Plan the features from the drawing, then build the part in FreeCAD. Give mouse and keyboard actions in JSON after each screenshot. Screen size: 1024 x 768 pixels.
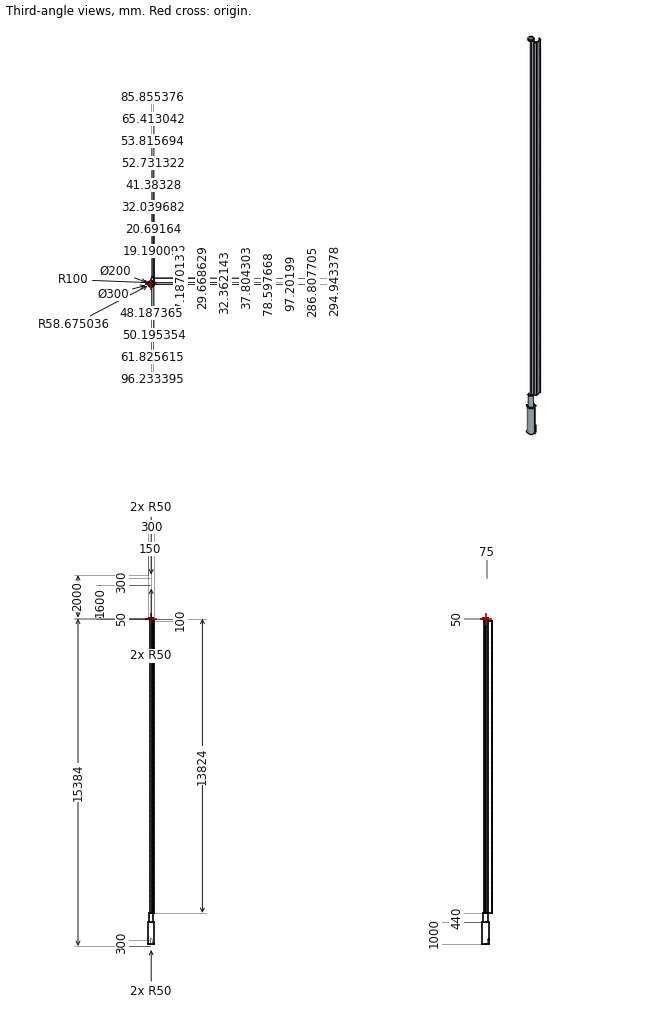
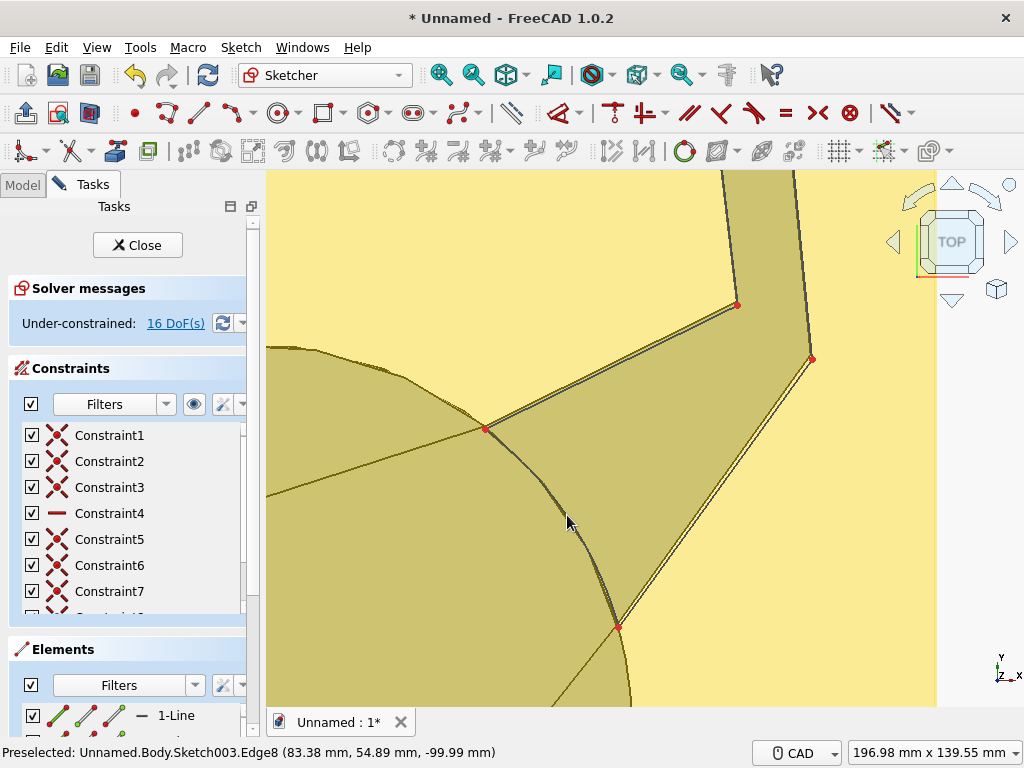
{"action": "scroll", "coordinate": [592, 548], "scroll_direction": "down", "scroll_amount": 7}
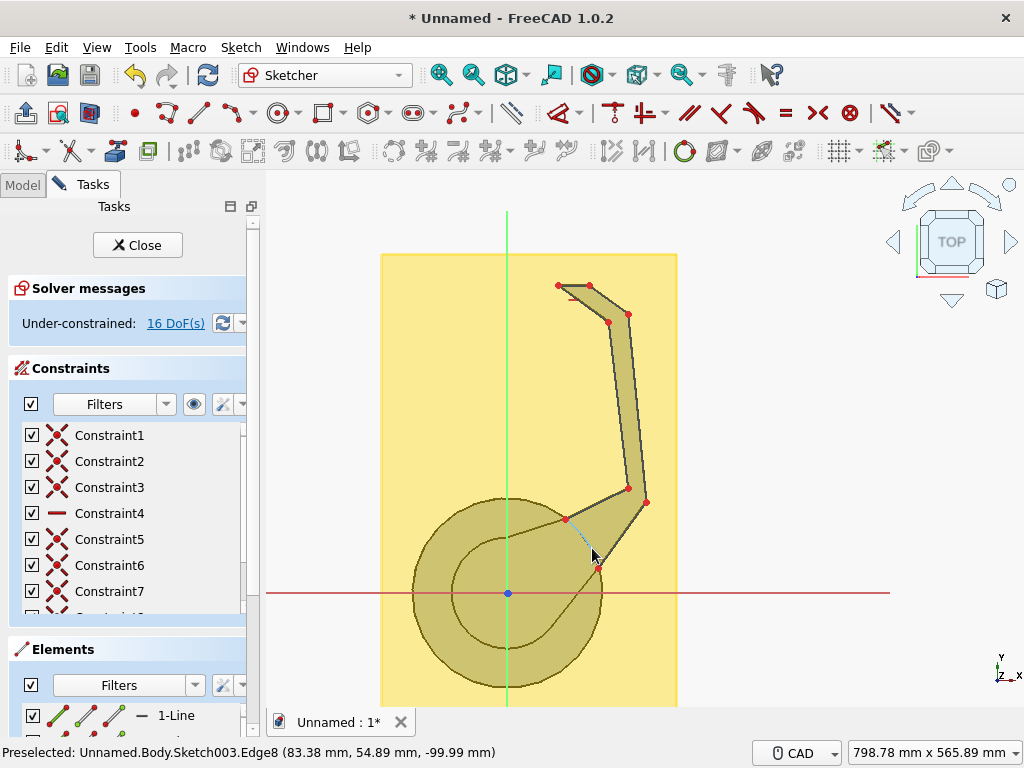
{"action": "left_click_drag", "start_coordinate": [497, 583], "coordinate": [519, 603]}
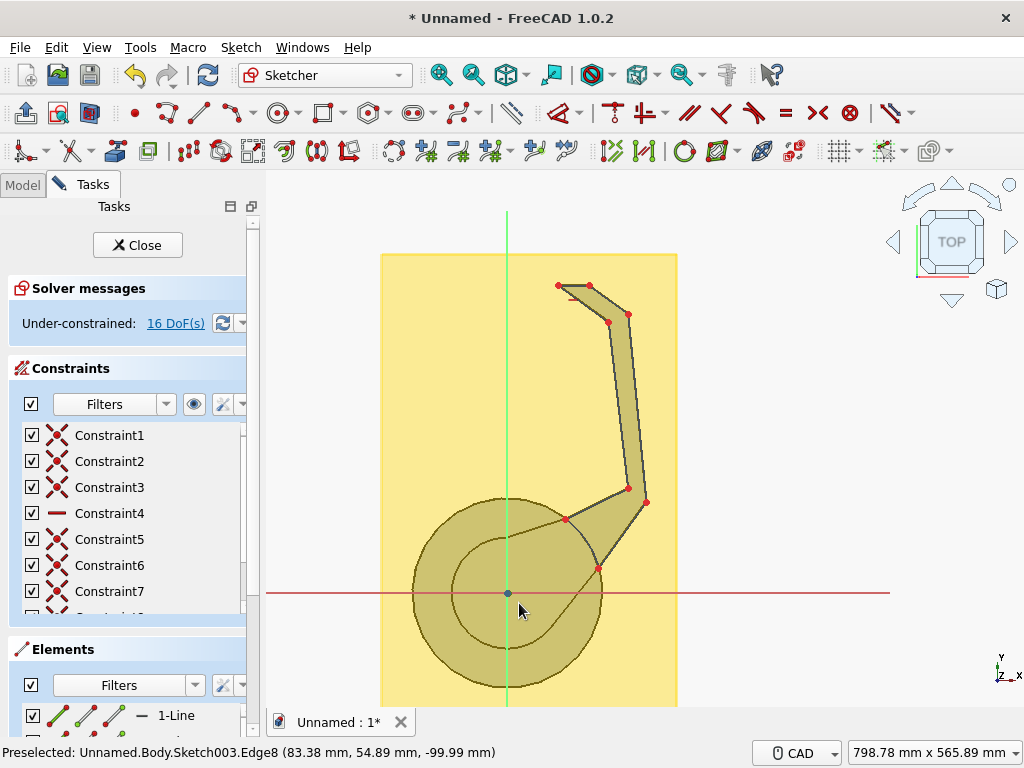
{"action": "left_click", "coordinate": [614, 114]}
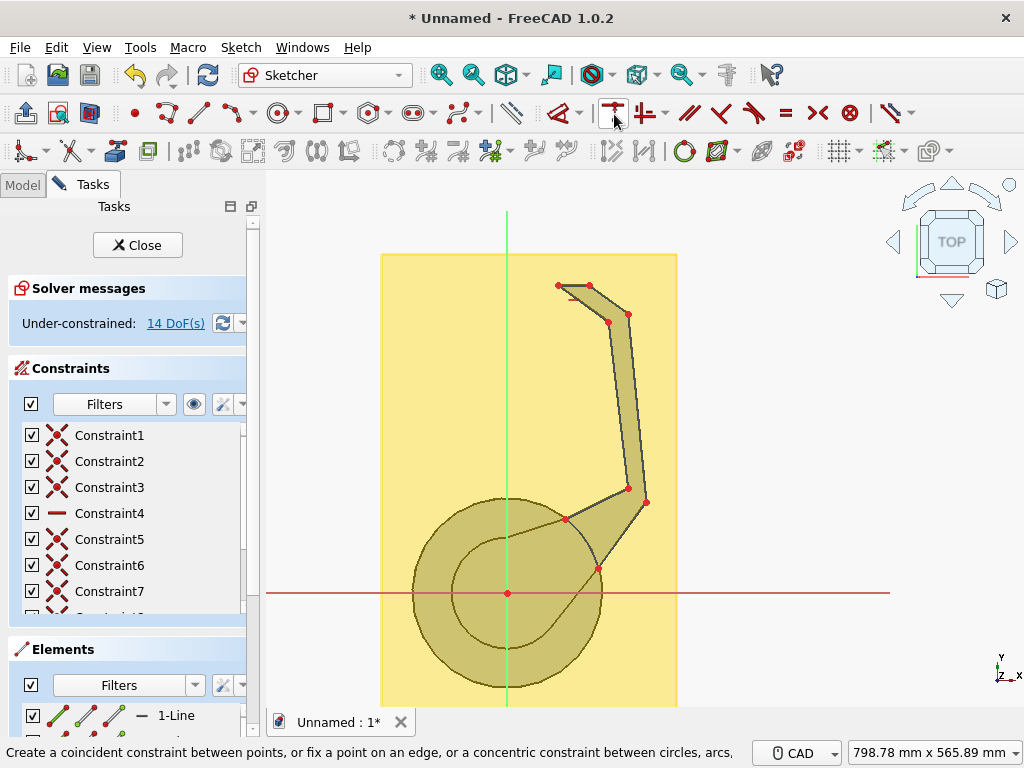
{"action": "left_click", "coordinate": [558, 114]}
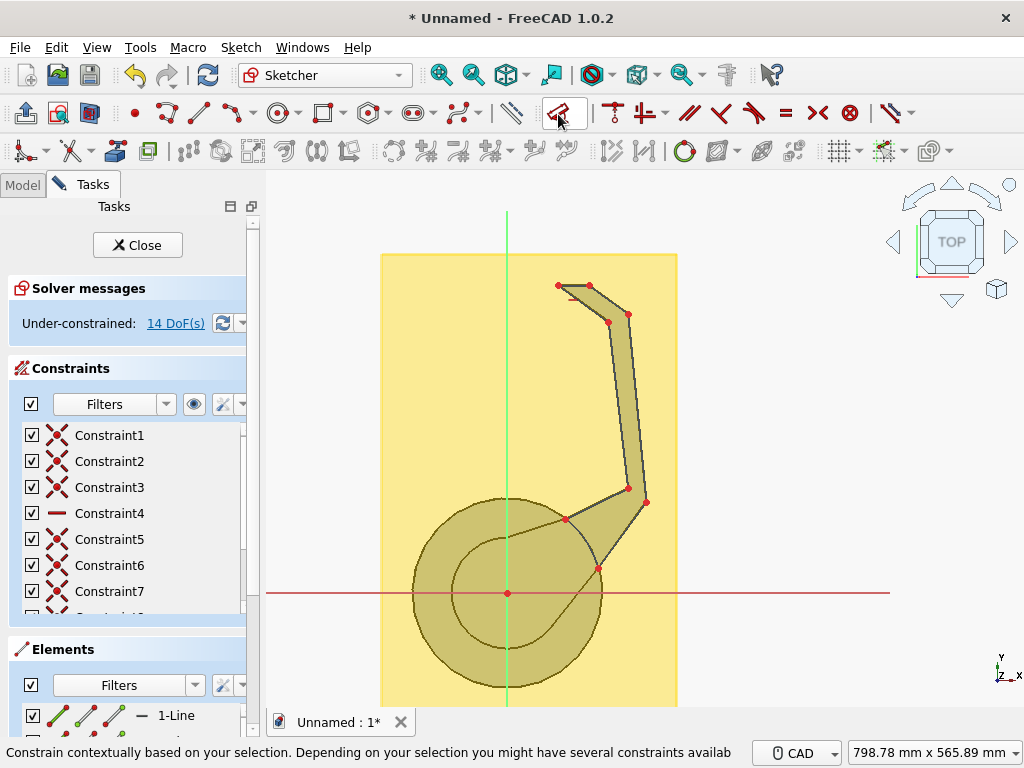
{"action": "left_click", "coordinate": [592, 551]}
{"action": "left_click", "coordinate": [580, 489]}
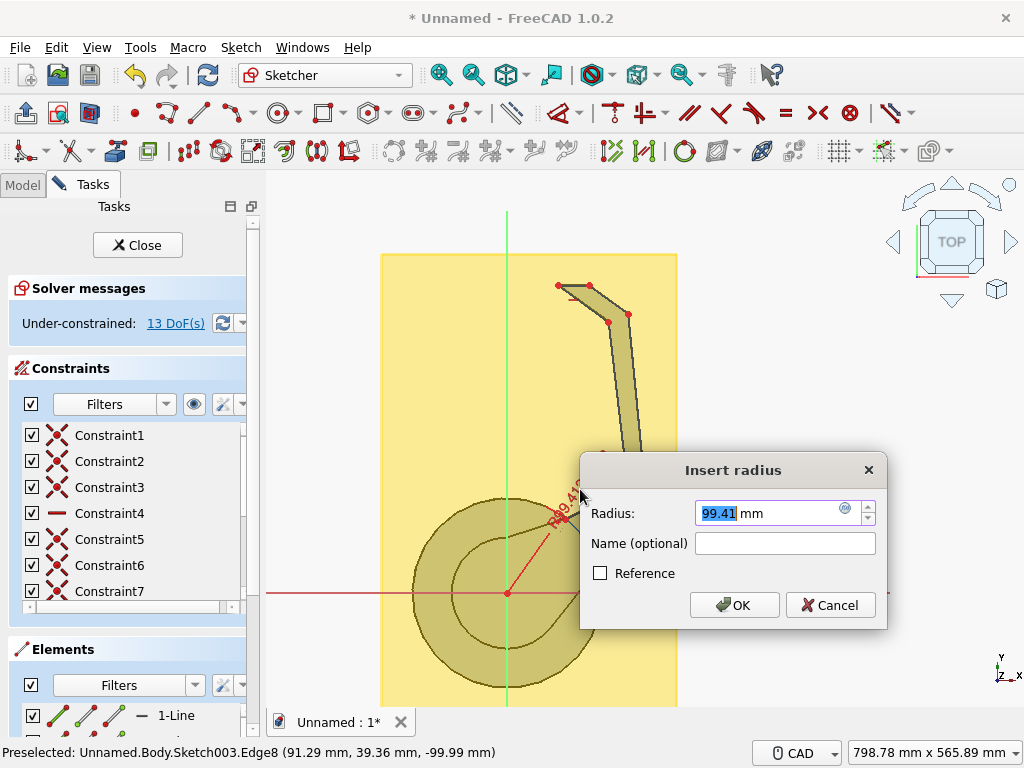
{"action": "type", "text": "100"}
{"action": "key", "text": "Return"}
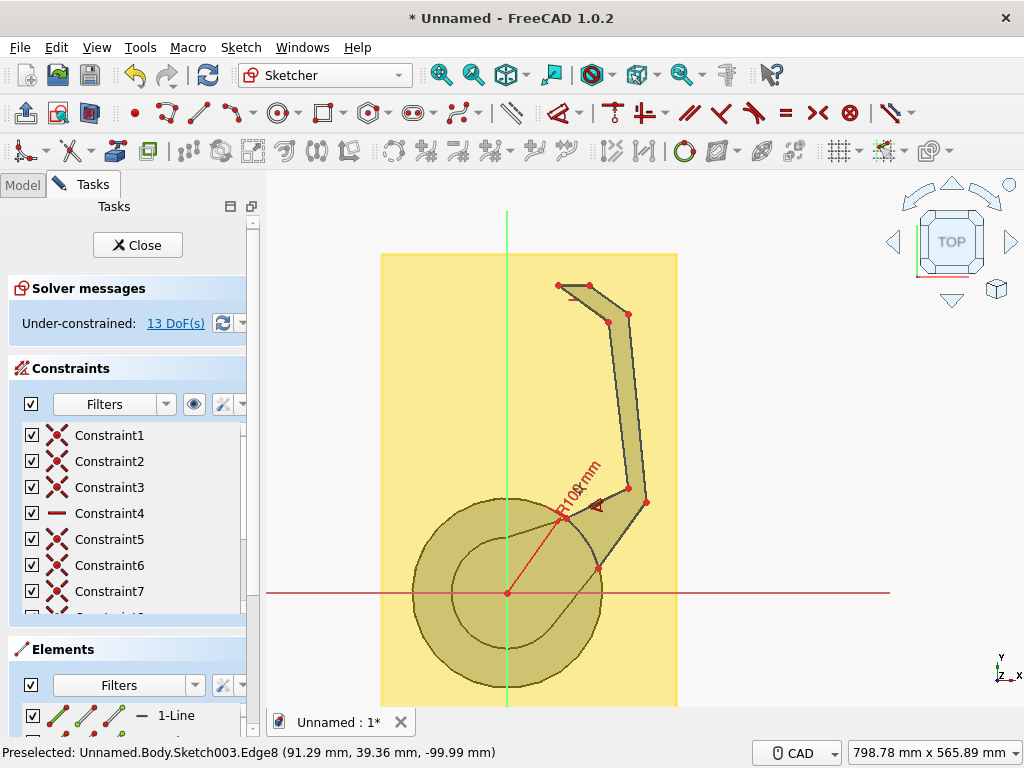
{"action": "scroll", "coordinate": [580, 286], "scroll_direction": "up", "scroll_amount": 3}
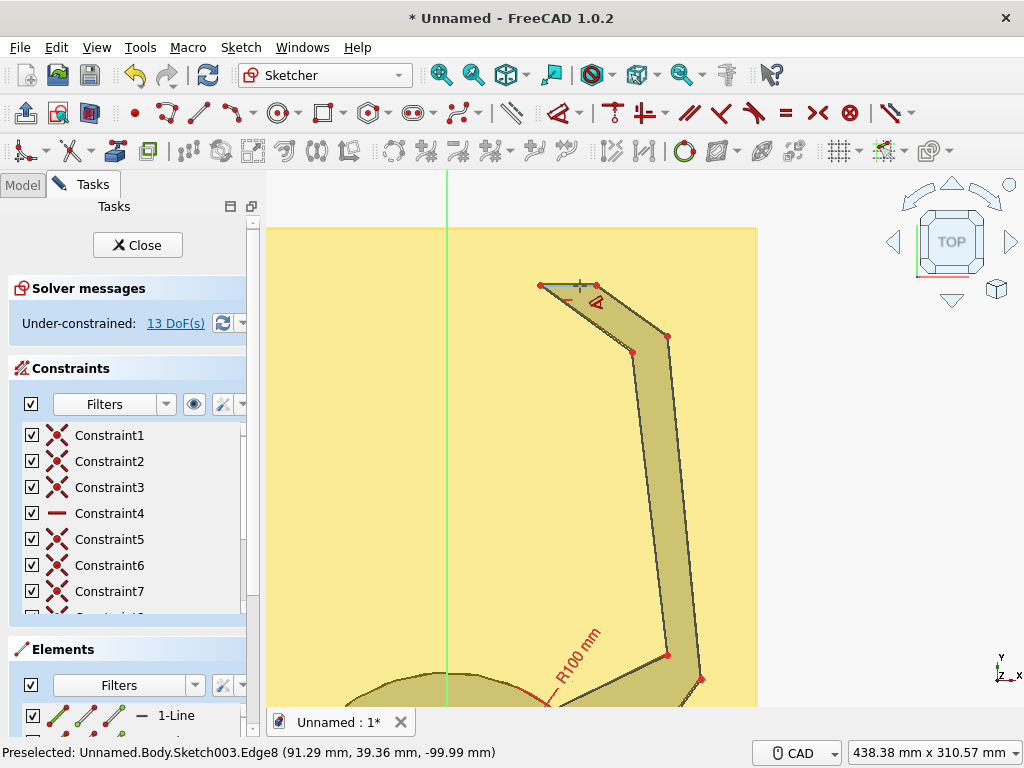
{"action": "left_click", "coordinate": [580, 286]}
{"action": "left_click", "coordinate": [569, 252]}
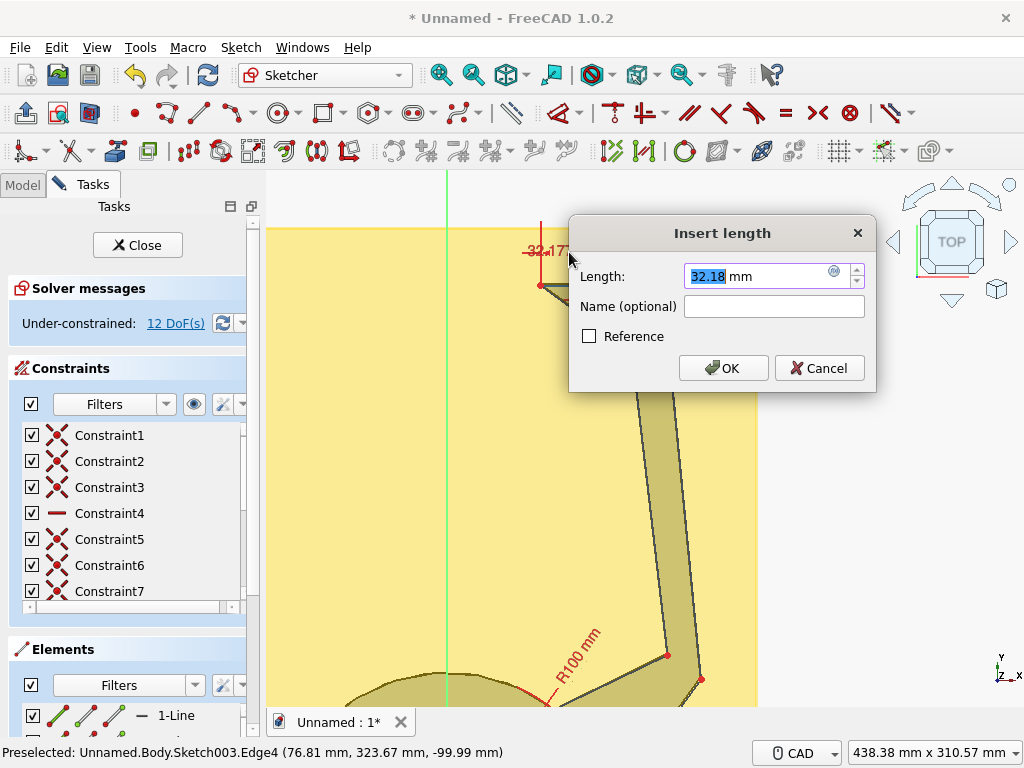
{"action": "type", "text": "32.039682"}
{"action": "key", "text": "Return"}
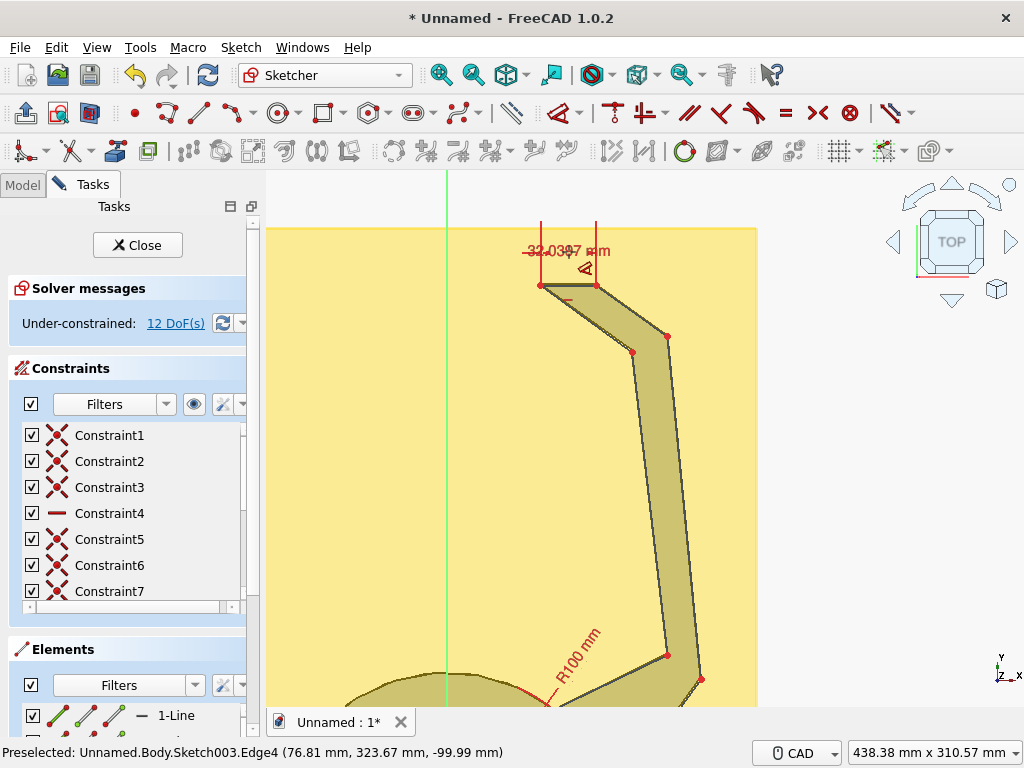
{"action": "scroll", "coordinate": [580, 285], "scroll_direction": "down", "scroll_amount": 3}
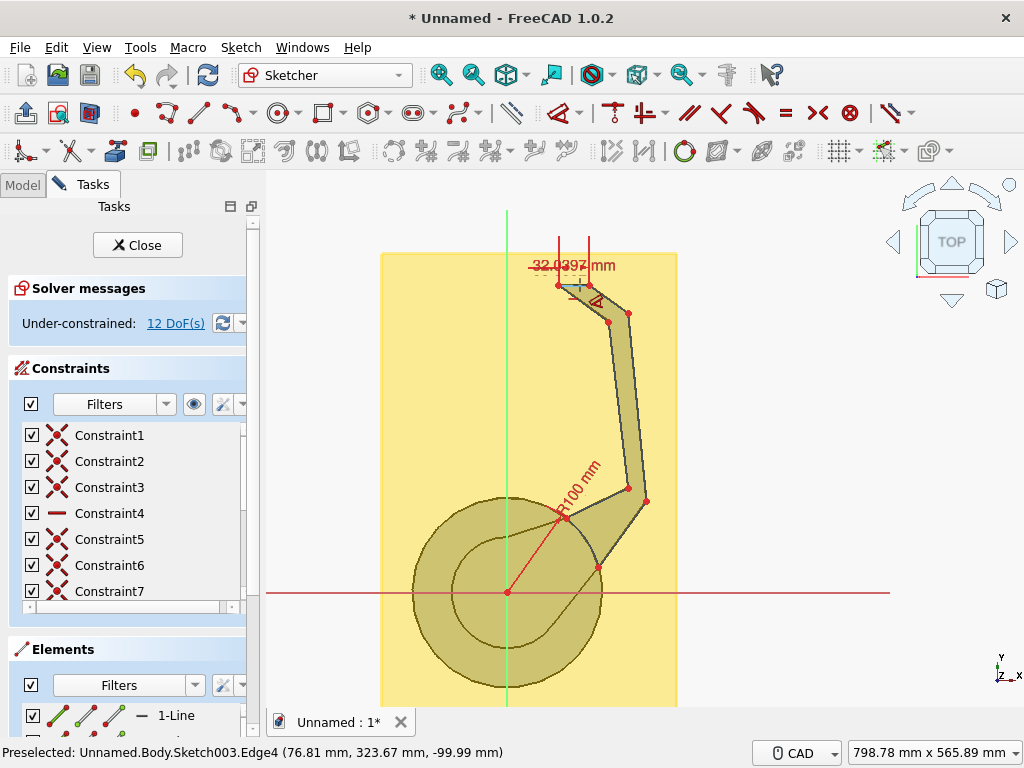
{"action": "left_click", "coordinate": [647, 502]}
{"action": "left_click", "coordinate": [681, 547]}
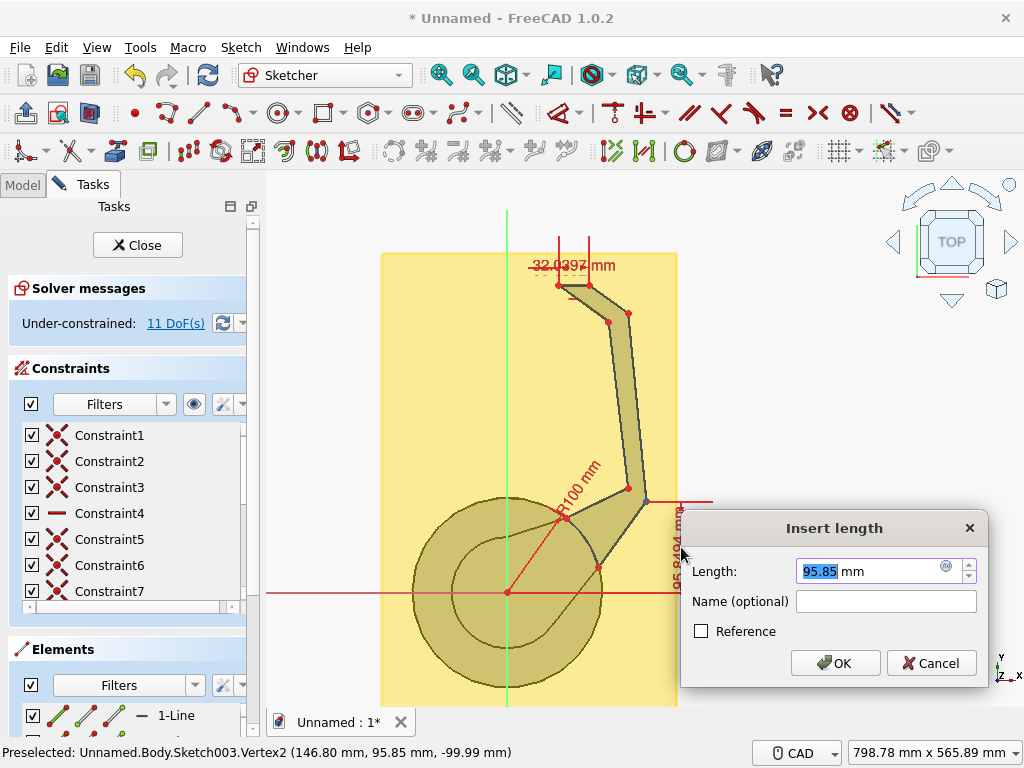
{"action": "type", "text": "97.20199"}
{"action": "key", "text": "Return"}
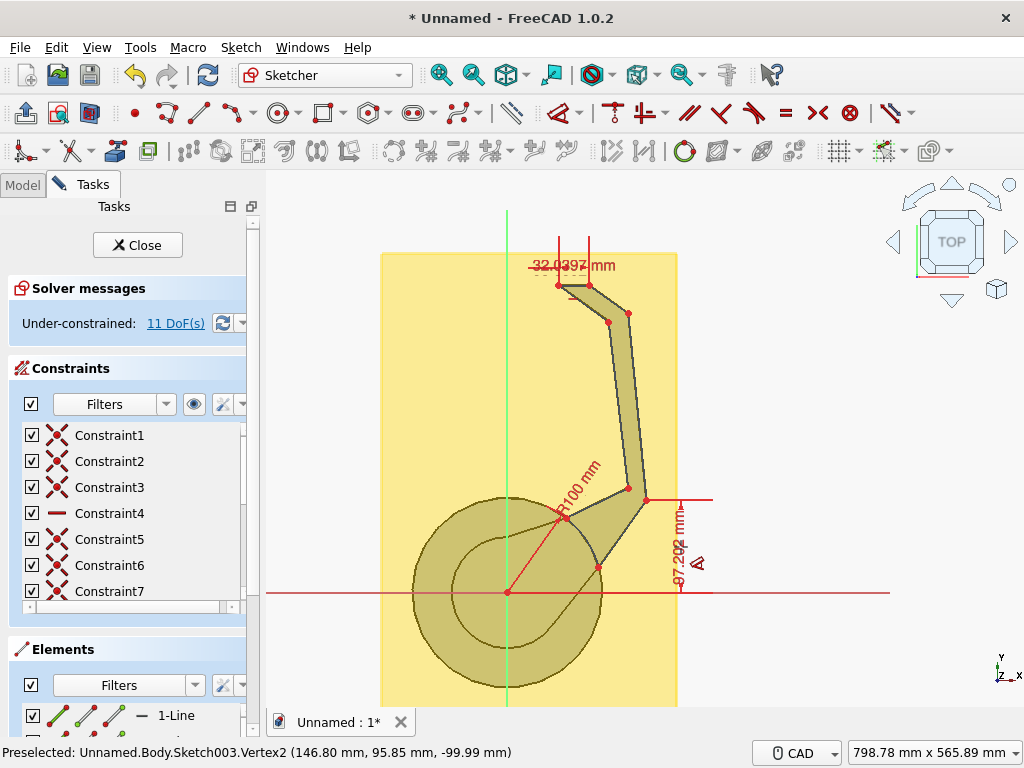
{"action": "left_click", "coordinate": [617, 305]}
{"action": "left_click", "coordinate": [595, 348]}